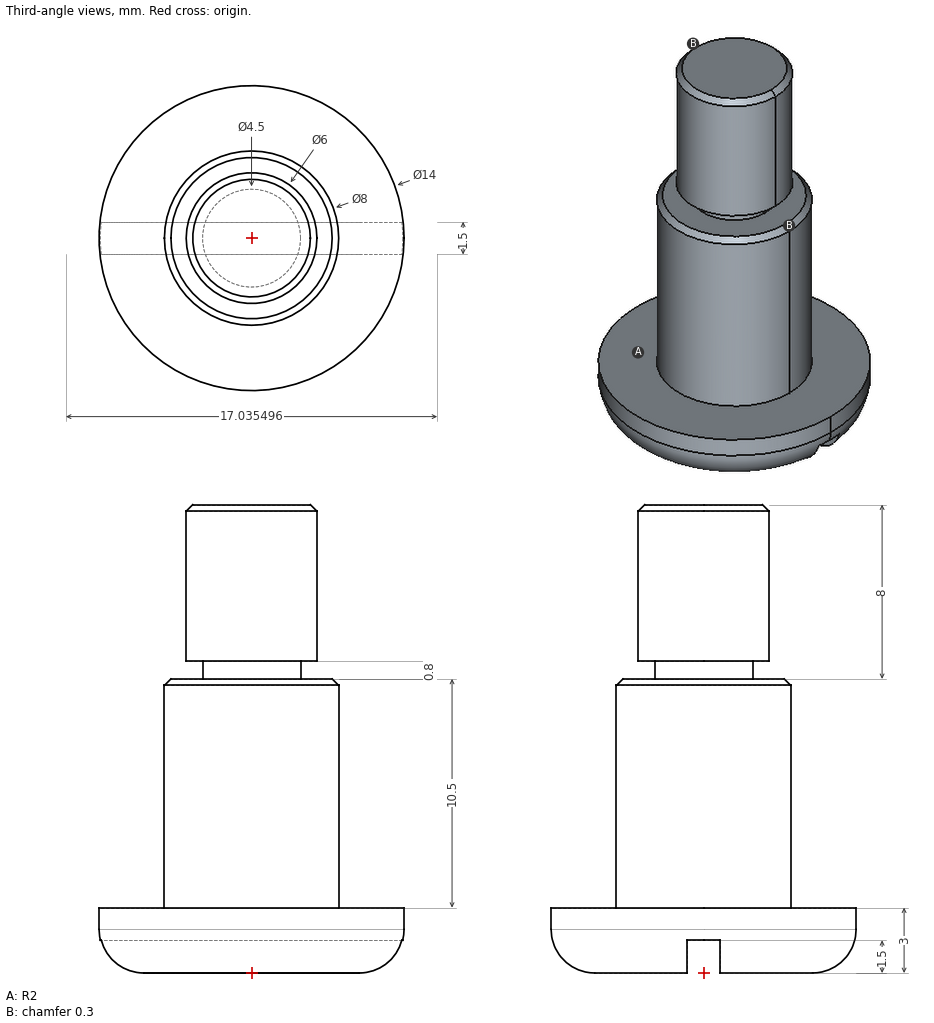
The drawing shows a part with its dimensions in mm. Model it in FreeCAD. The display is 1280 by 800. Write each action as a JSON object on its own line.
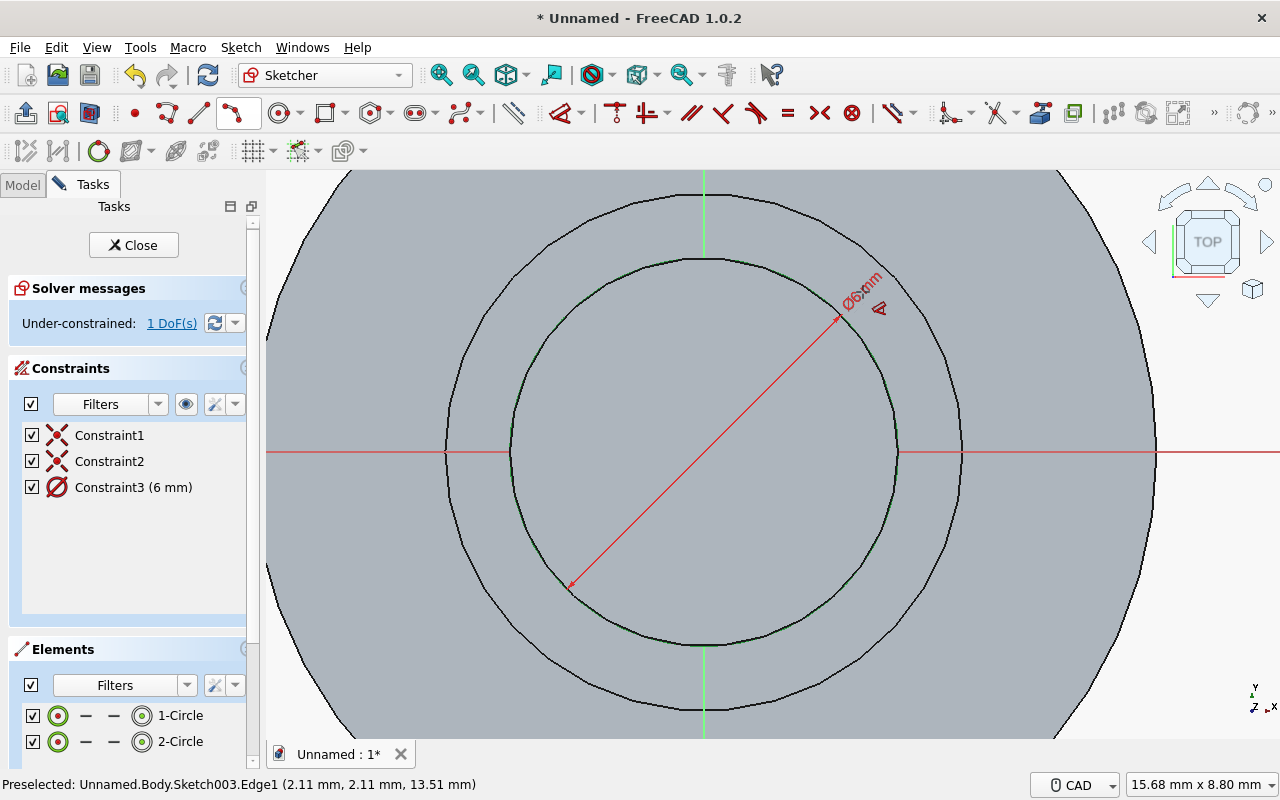
{"action": "left_click", "coordinate": [806, 349]}
{"action": "left_click", "coordinate": [829, 326]}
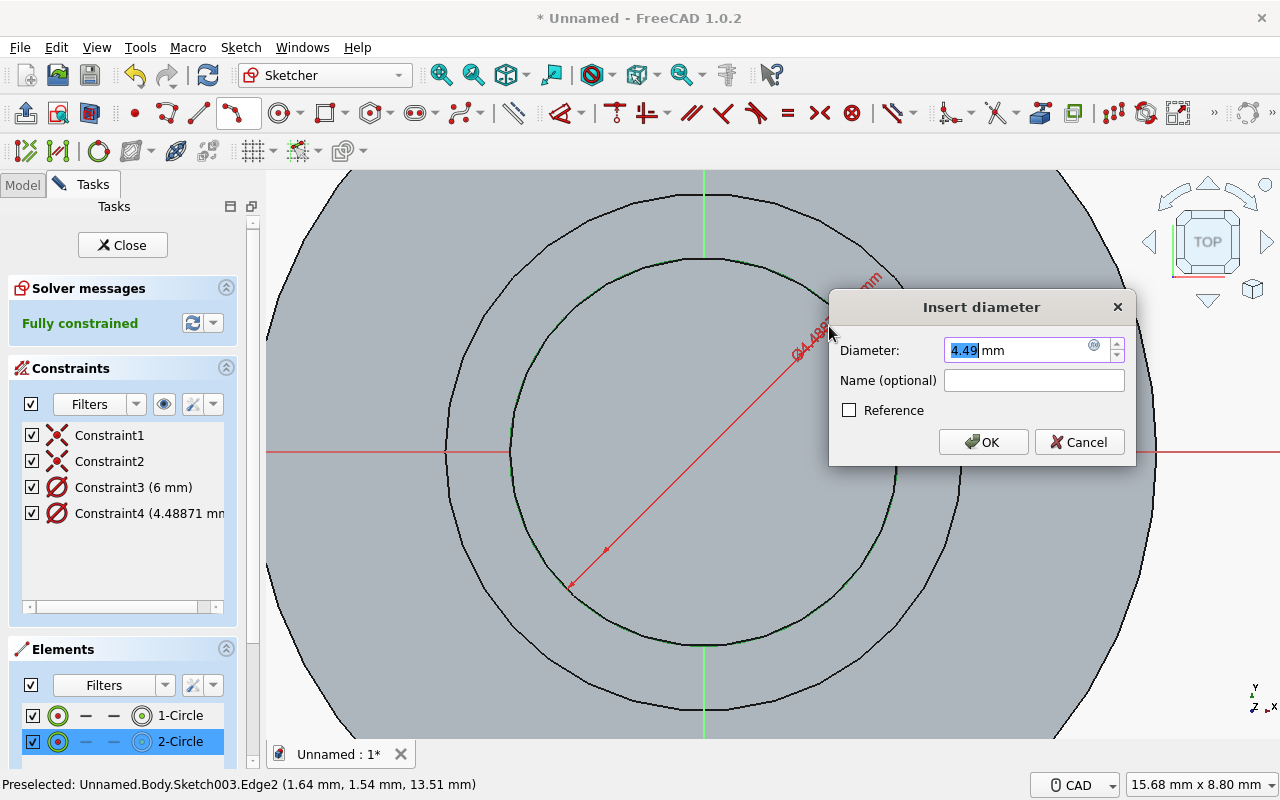
{"action": "type", "text": "4.5"}
{"action": "key", "text": "Return"}
{"action": "key", "text": "Escape"}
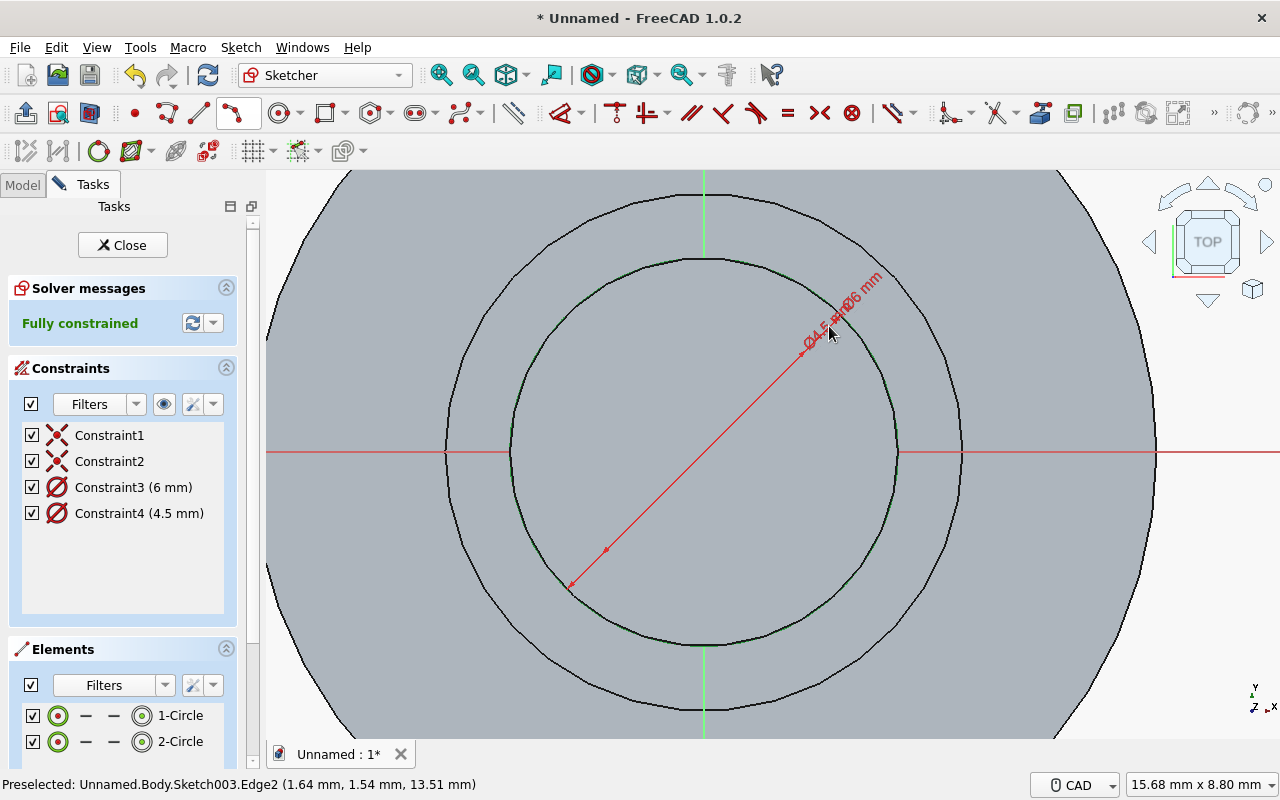
{"action": "left_click", "coordinate": [123, 245]}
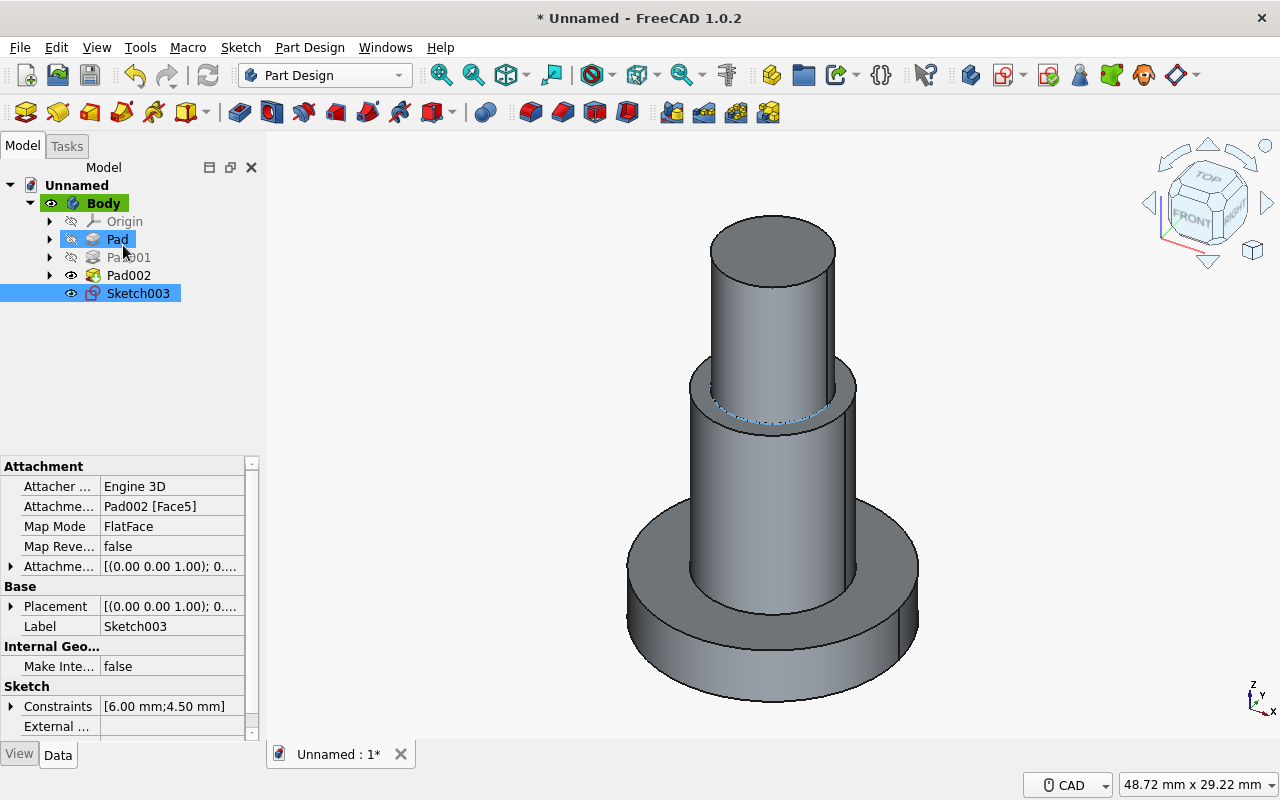
{"action": "left_click", "coordinate": [240, 112]}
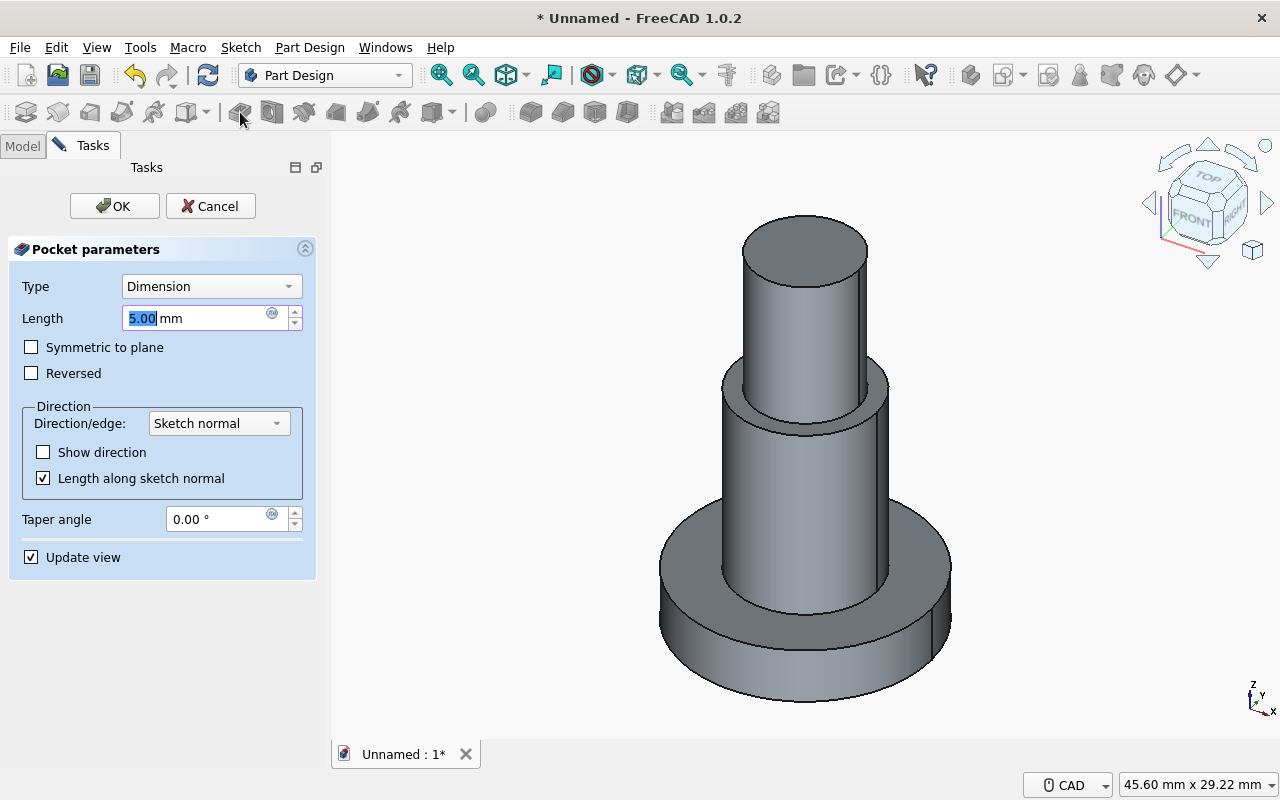
{"action": "type", "text": "0.8"}
{"action": "key", "text": "Tab"}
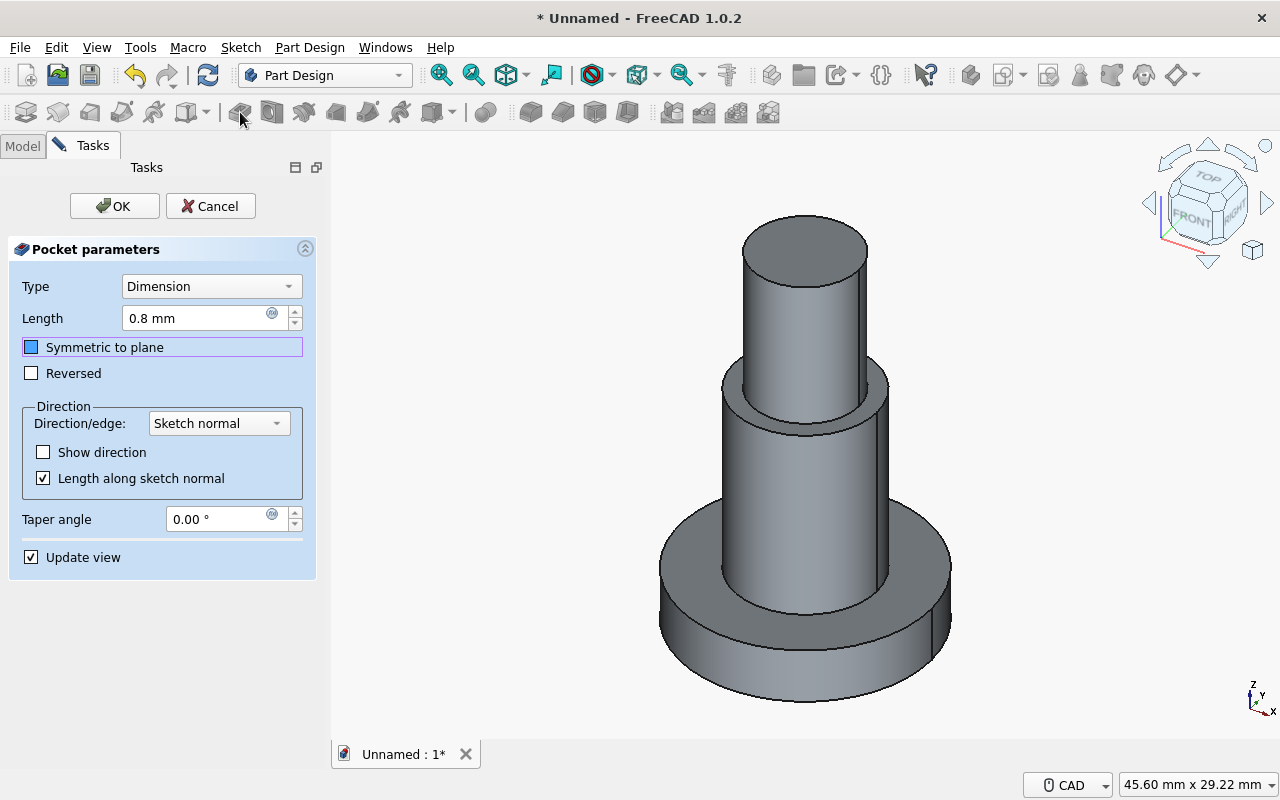
{"action": "left_click", "coordinate": [30, 373]}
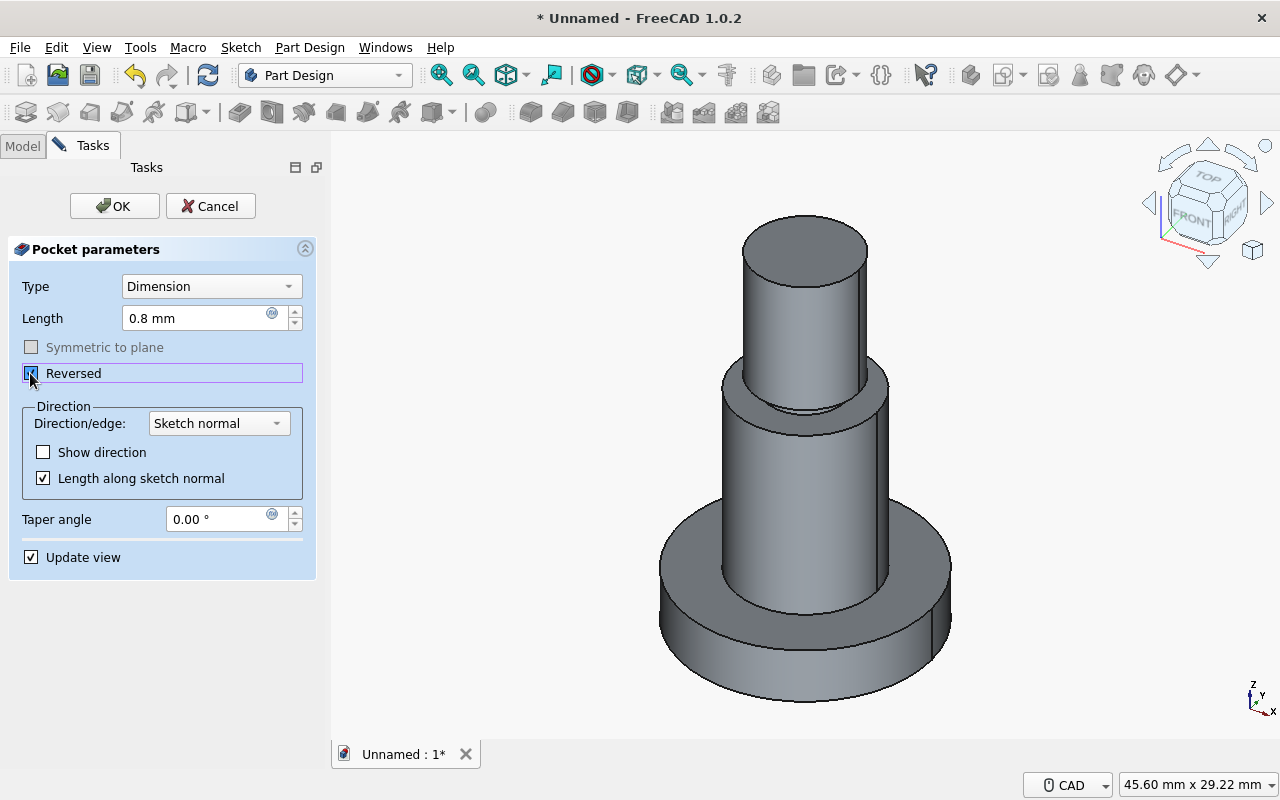
{"action": "left_click", "coordinate": [115, 206]}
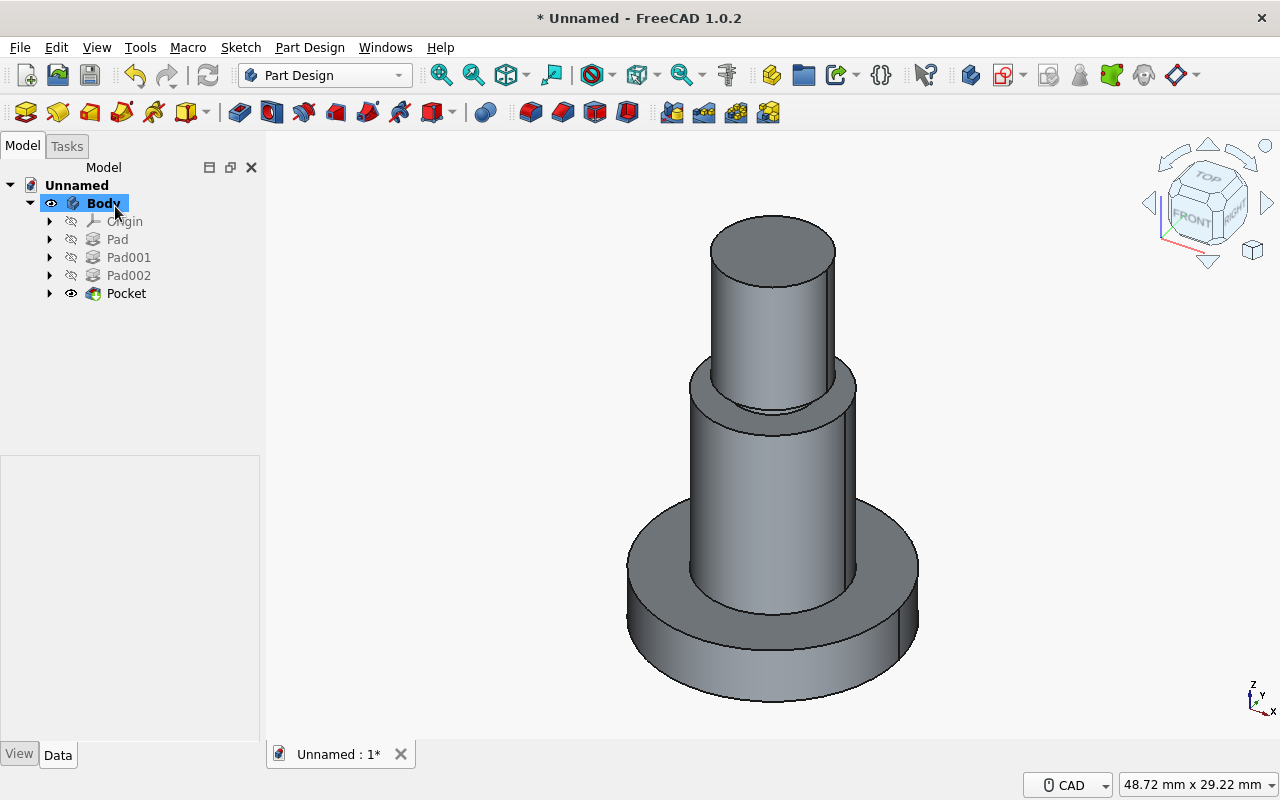
{"action": "key", "text": "0"}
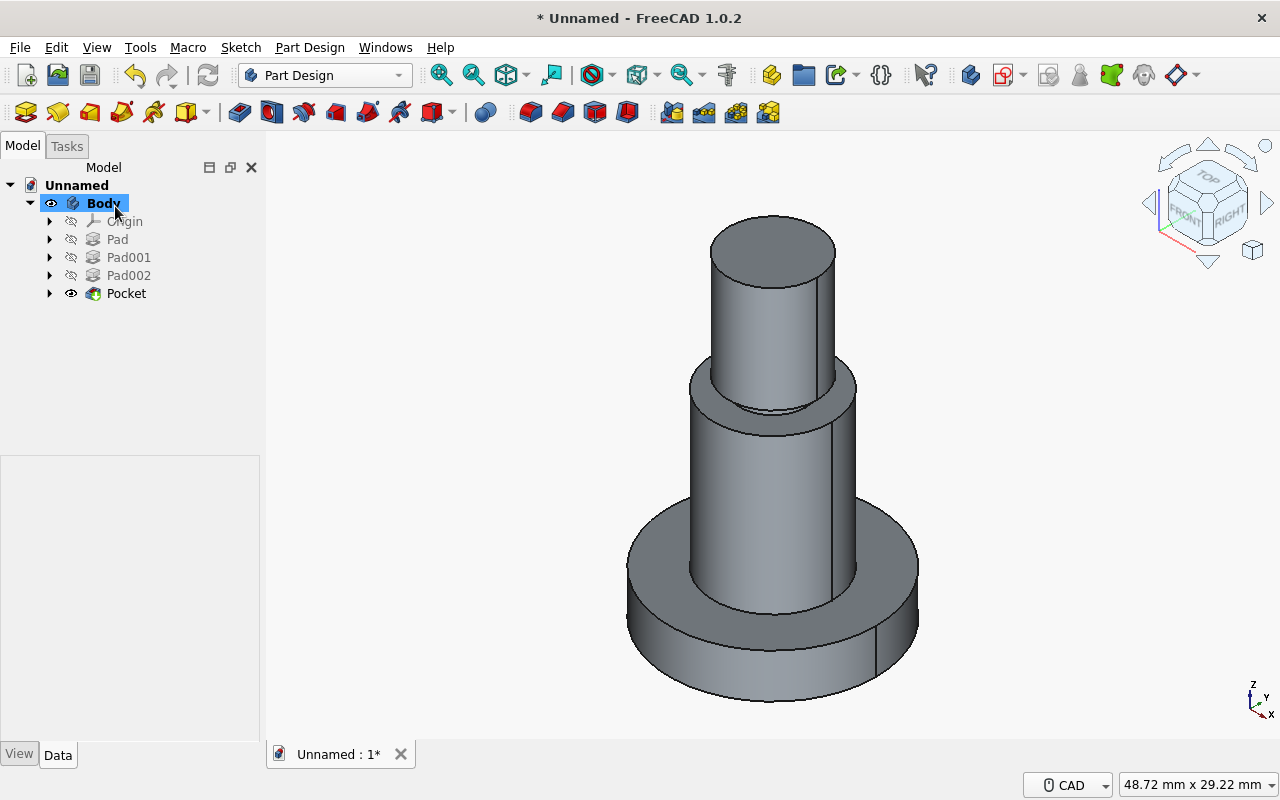
{"action": "key", "text": "2"}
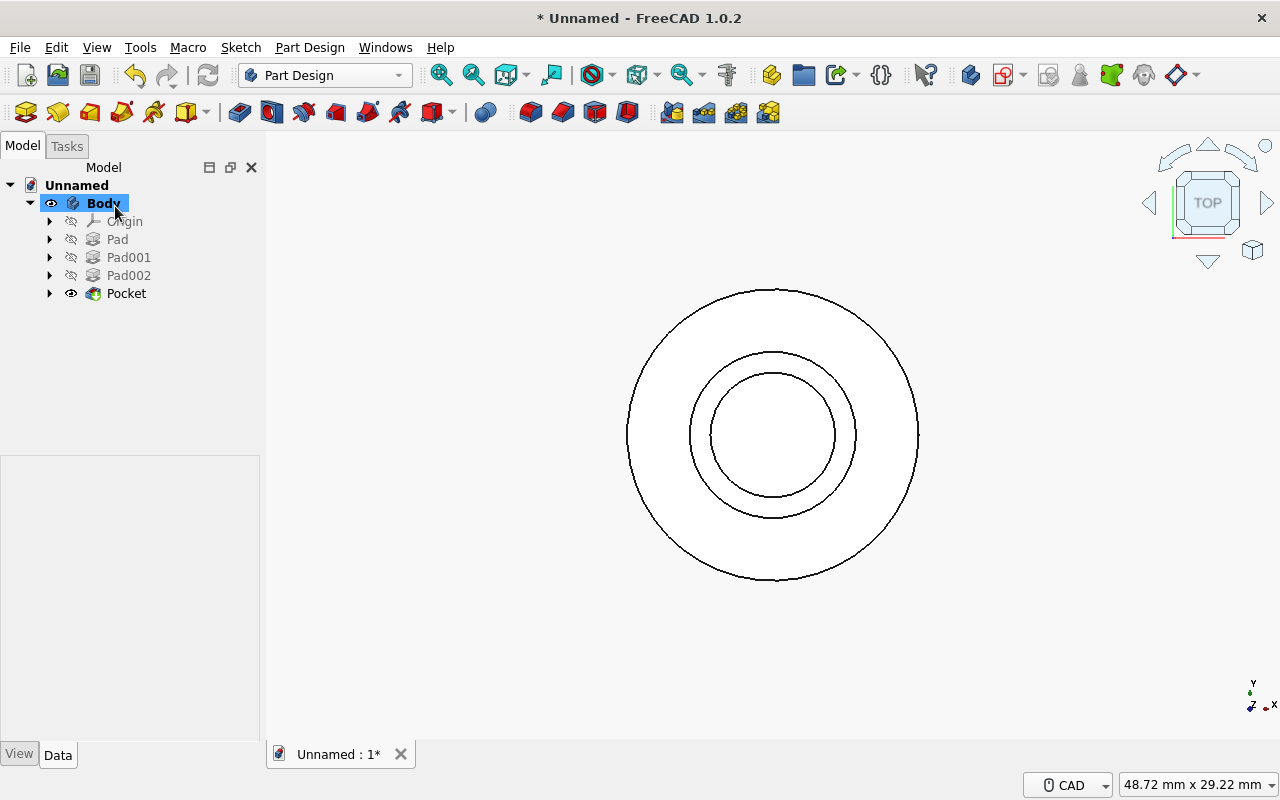
{"action": "key", "text": "1"}